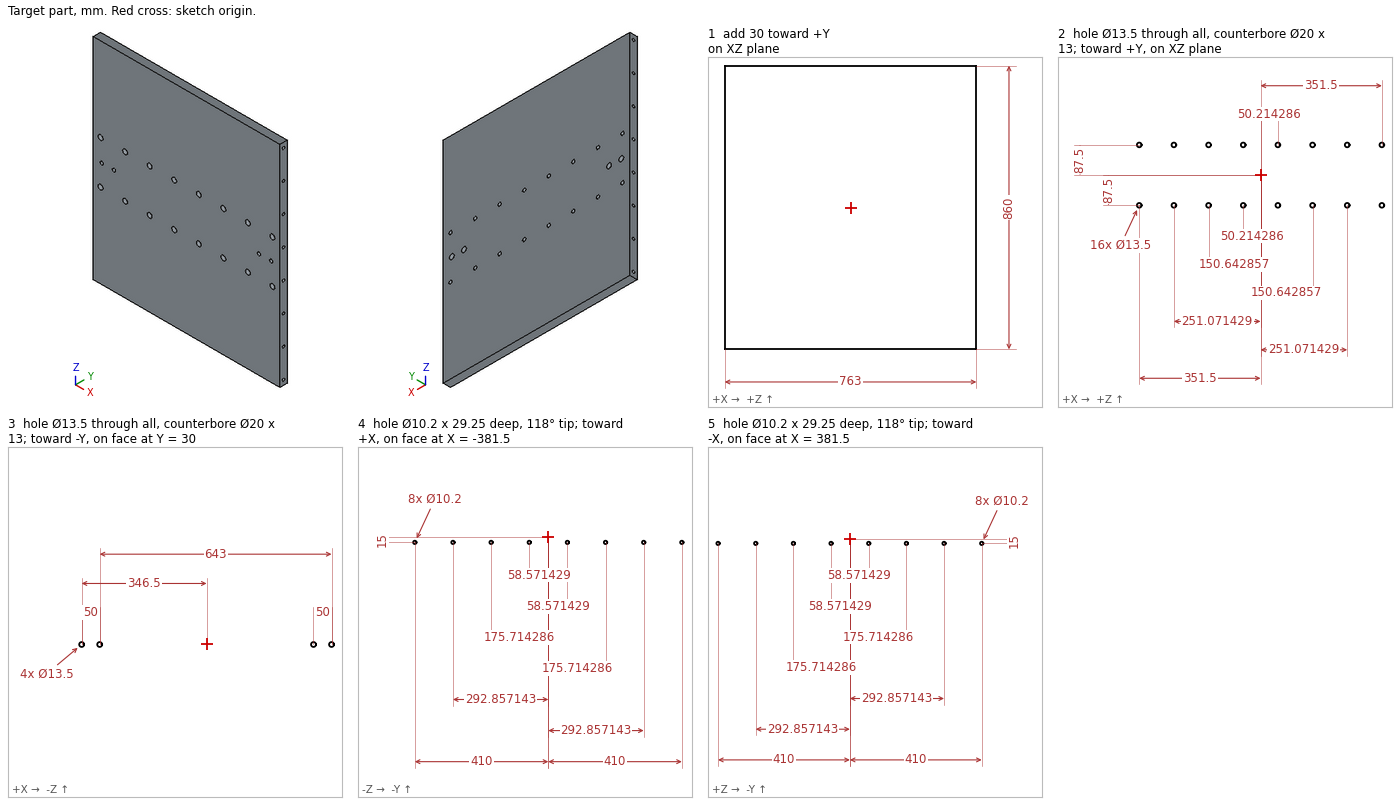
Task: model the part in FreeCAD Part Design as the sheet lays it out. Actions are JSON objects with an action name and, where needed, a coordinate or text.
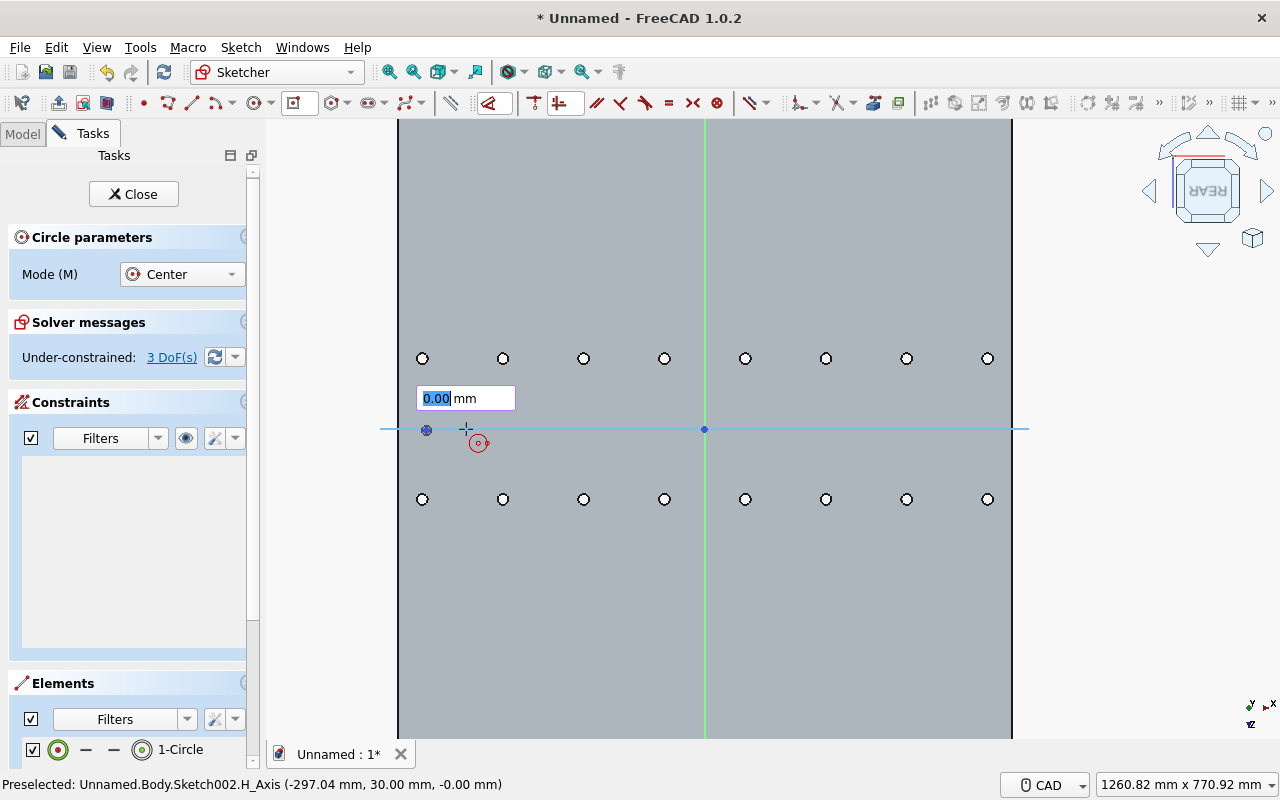
{"action": "scroll", "coordinate": [465, 434], "scroll_direction": "up", "scroll_amount": 6}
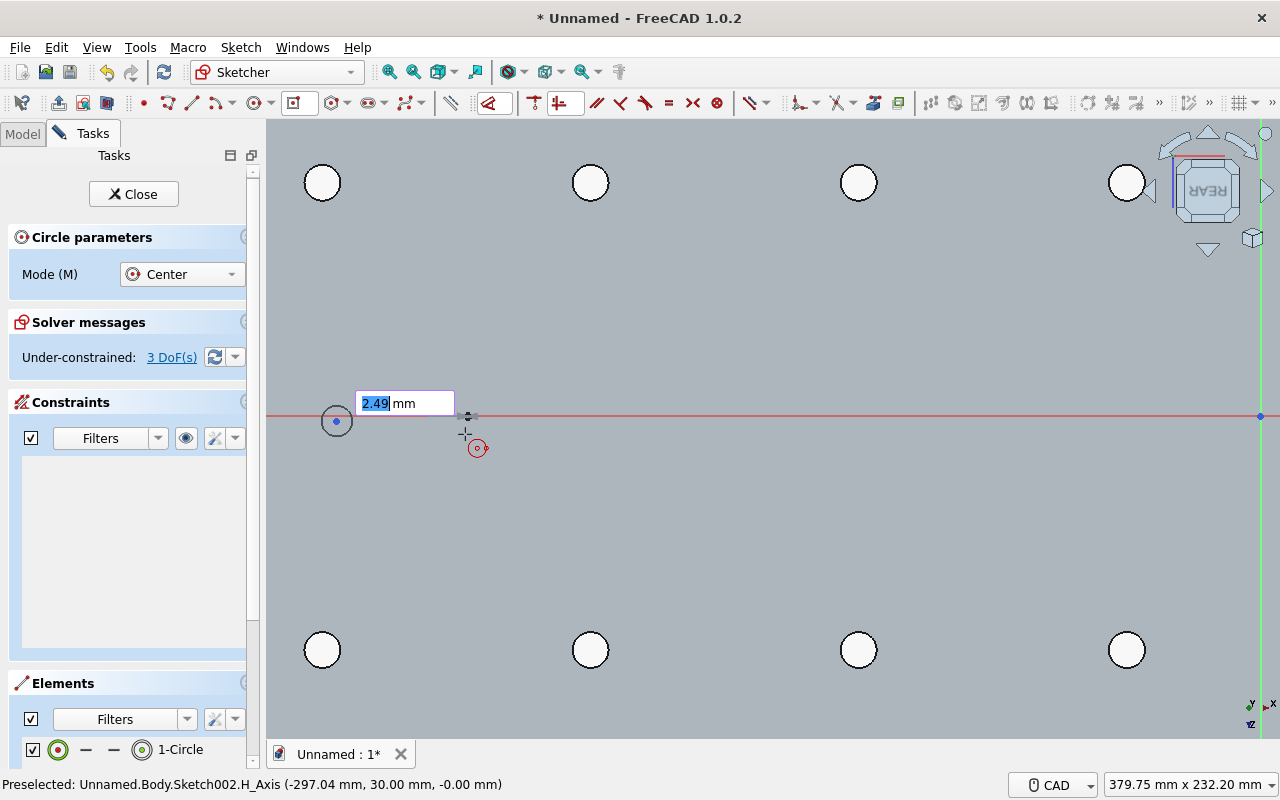
{"action": "left_click", "coordinate": [463, 433]}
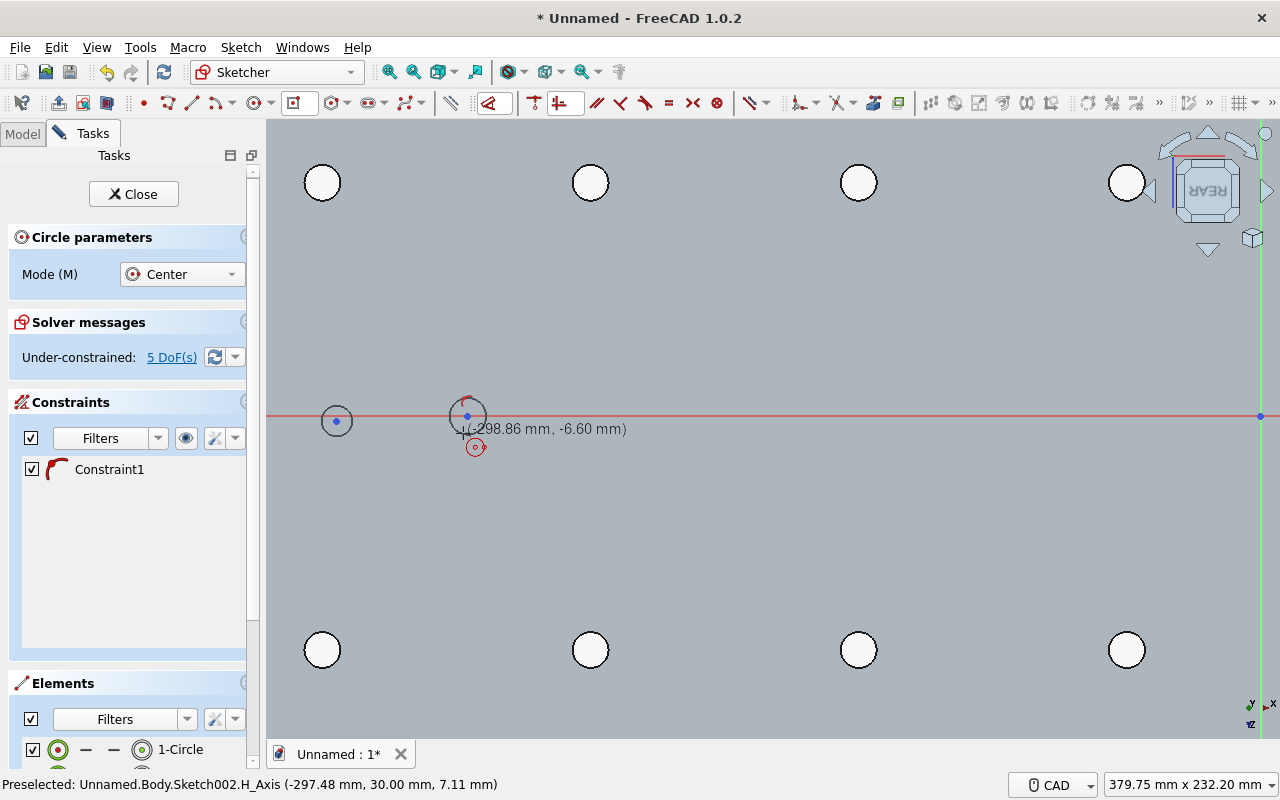
{"action": "scroll", "coordinate": [465, 434], "scroll_direction": "down", "scroll_amount": 6}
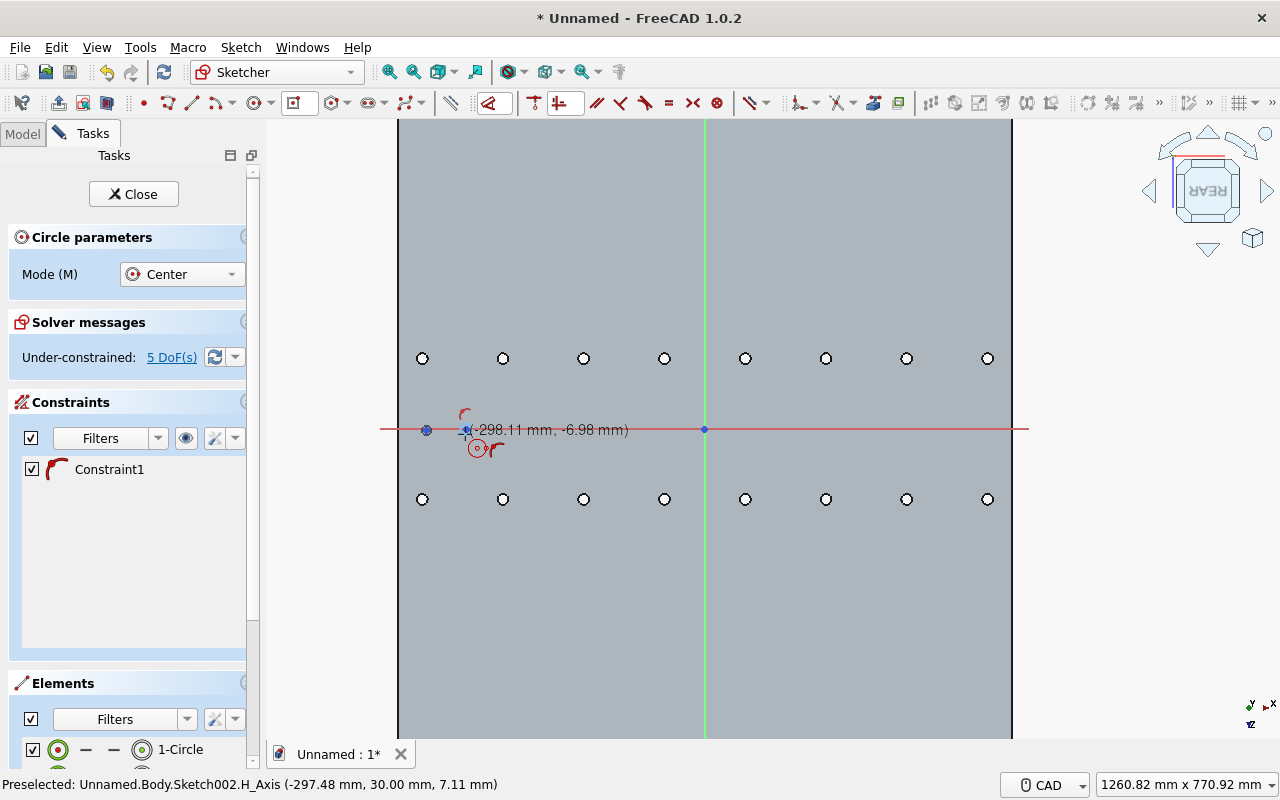
{"action": "scroll", "coordinate": [984, 429], "scroll_direction": "up", "scroll_amount": 8}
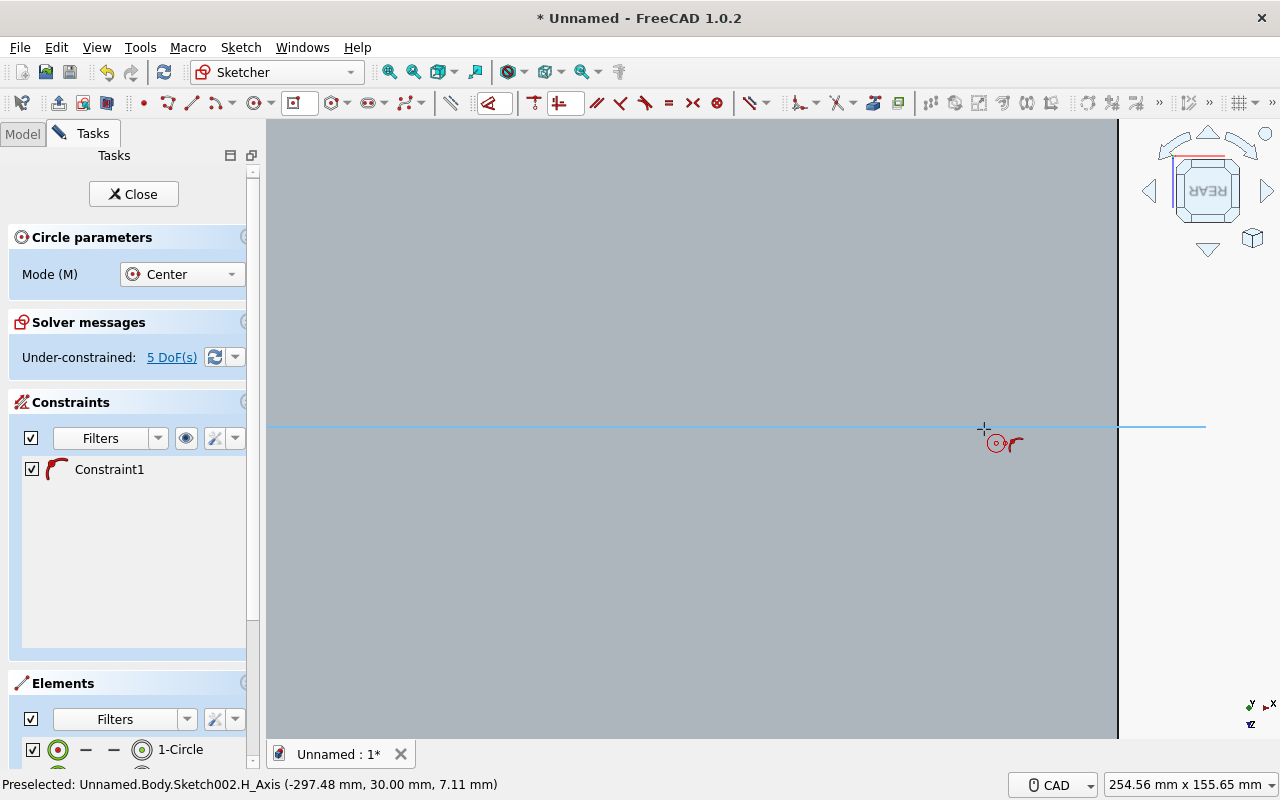
{"action": "scroll", "coordinate": [984, 429], "scroll_direction": "down", "scroll_amount": 8}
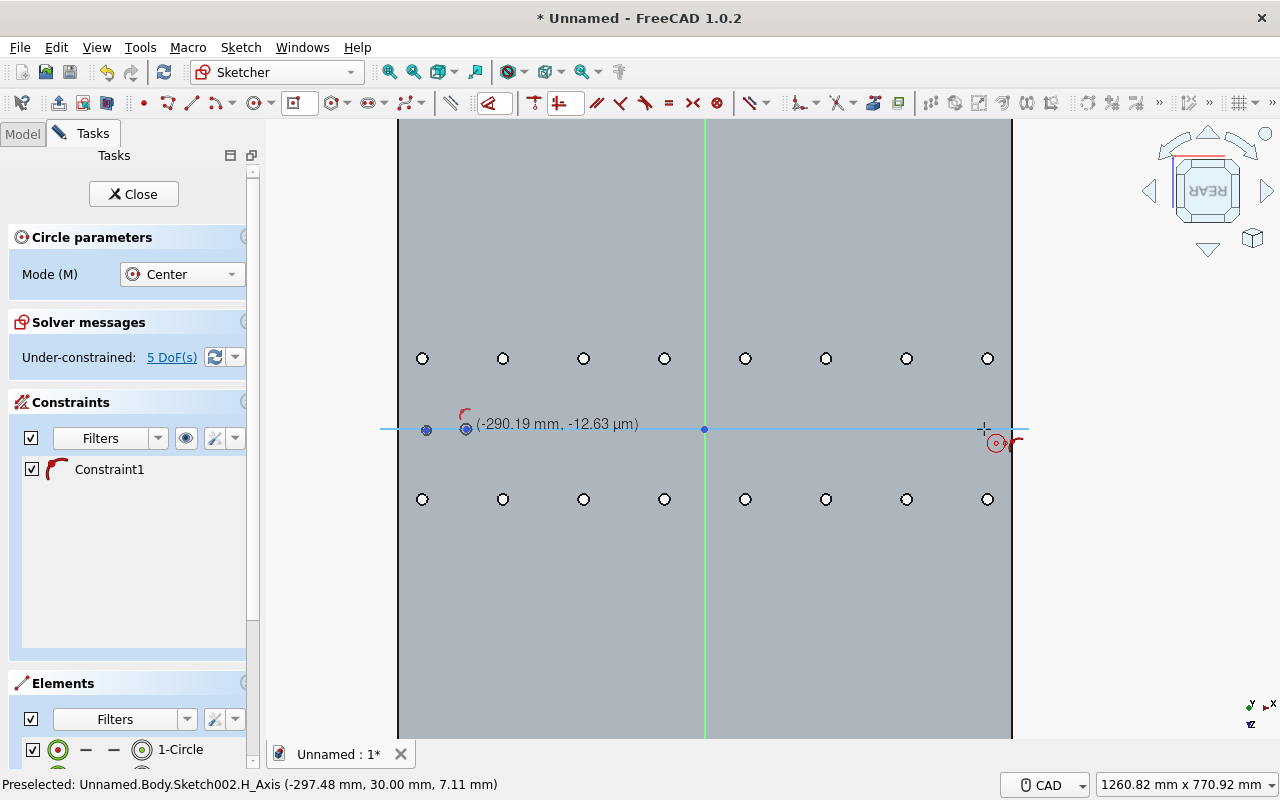
{"action": "left_click", "coordinate": [984, 429]}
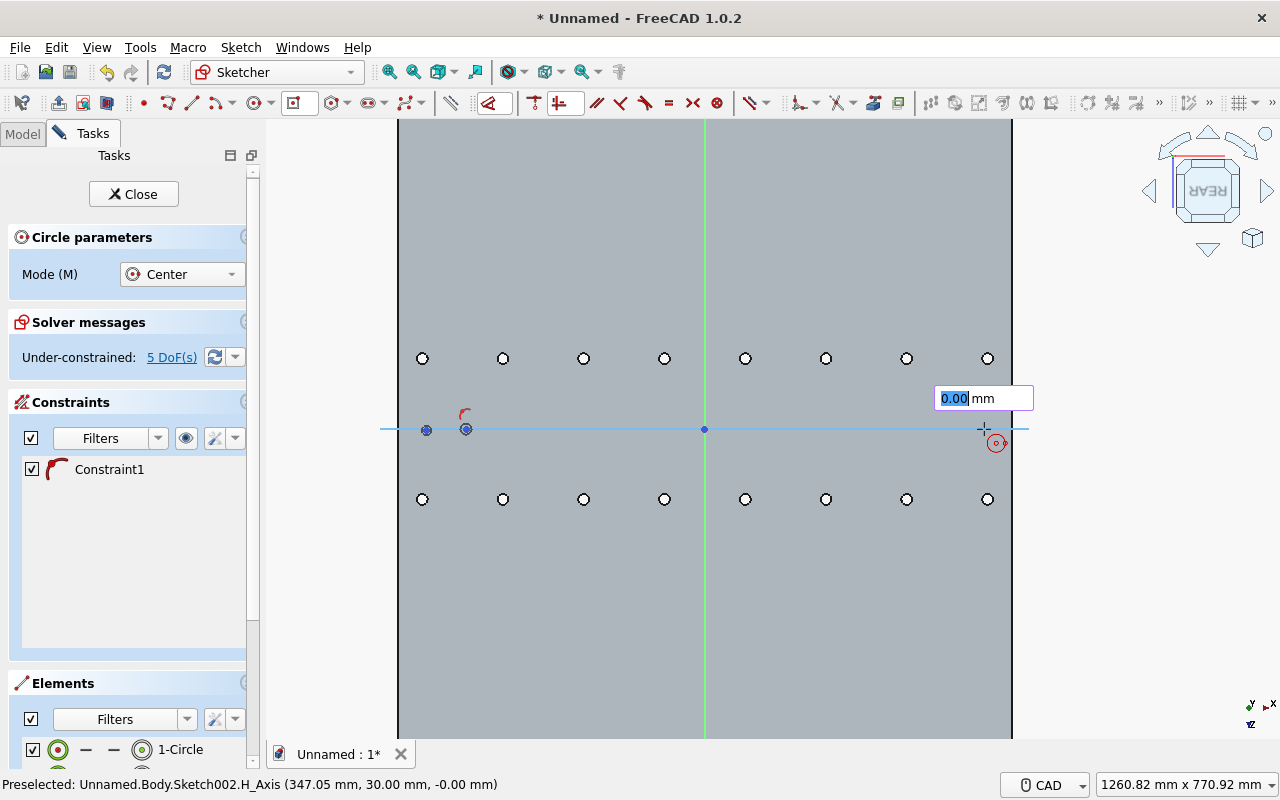
{"action": "scroll", "coordinate": [982, 434], "scroll_direction": "up", "scroll_amount": 6}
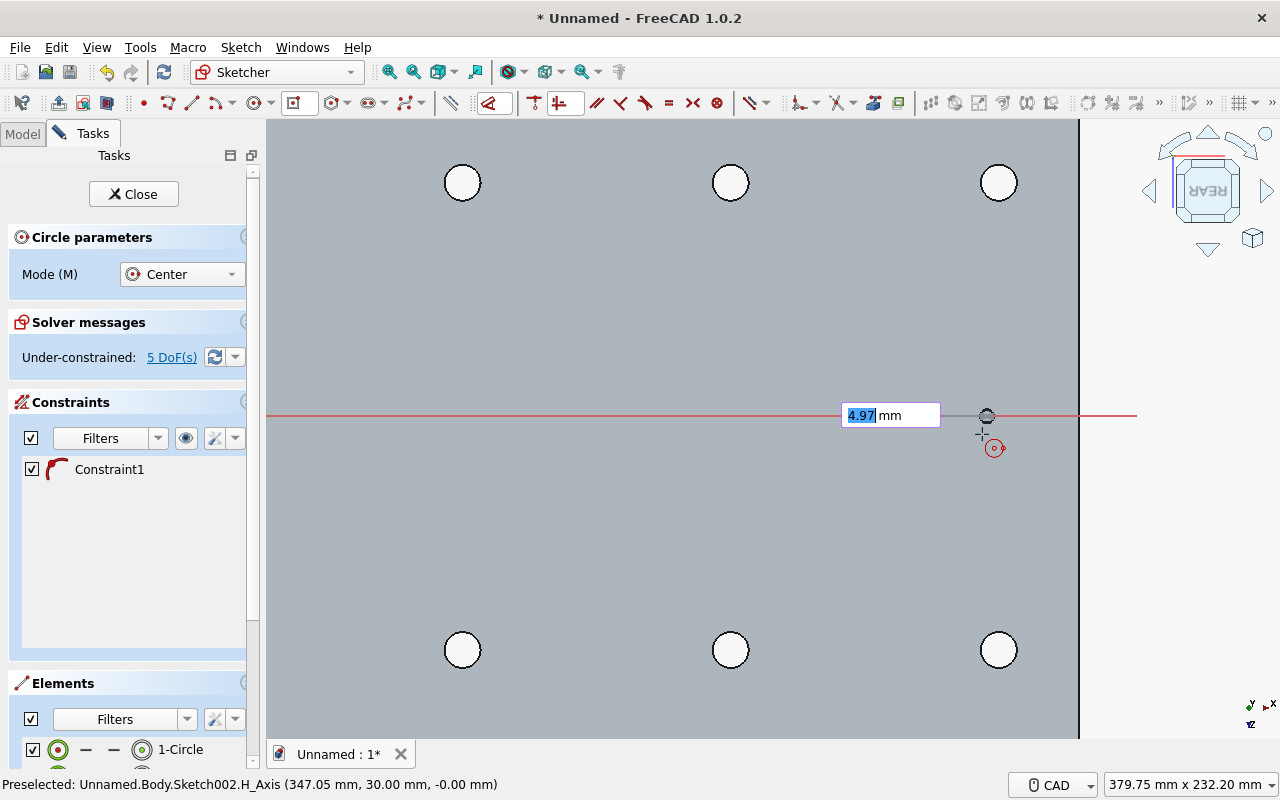
{"action": "left_click", "coordinate": [979, 433]}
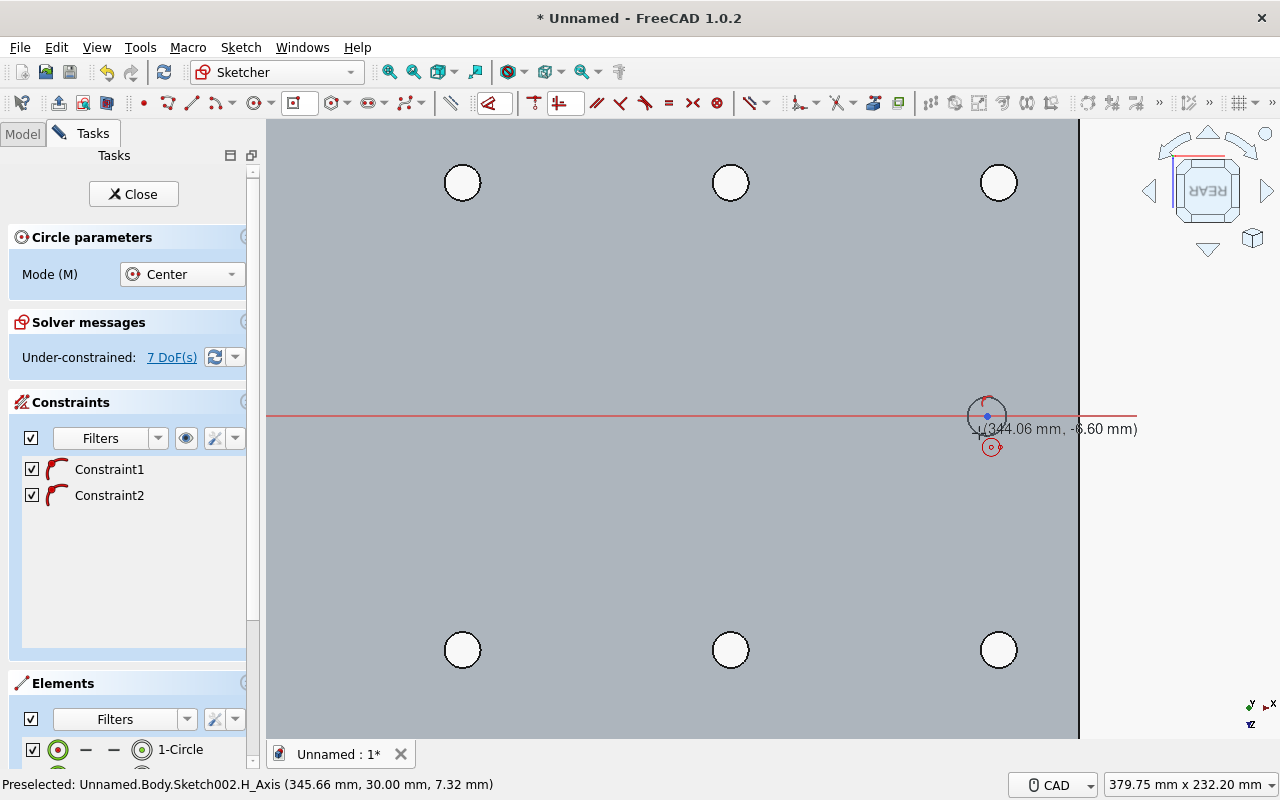
{"action": "scroll", "coordinate": [852, 416], "scroll_direction": "up", "scroll_amount": 2}